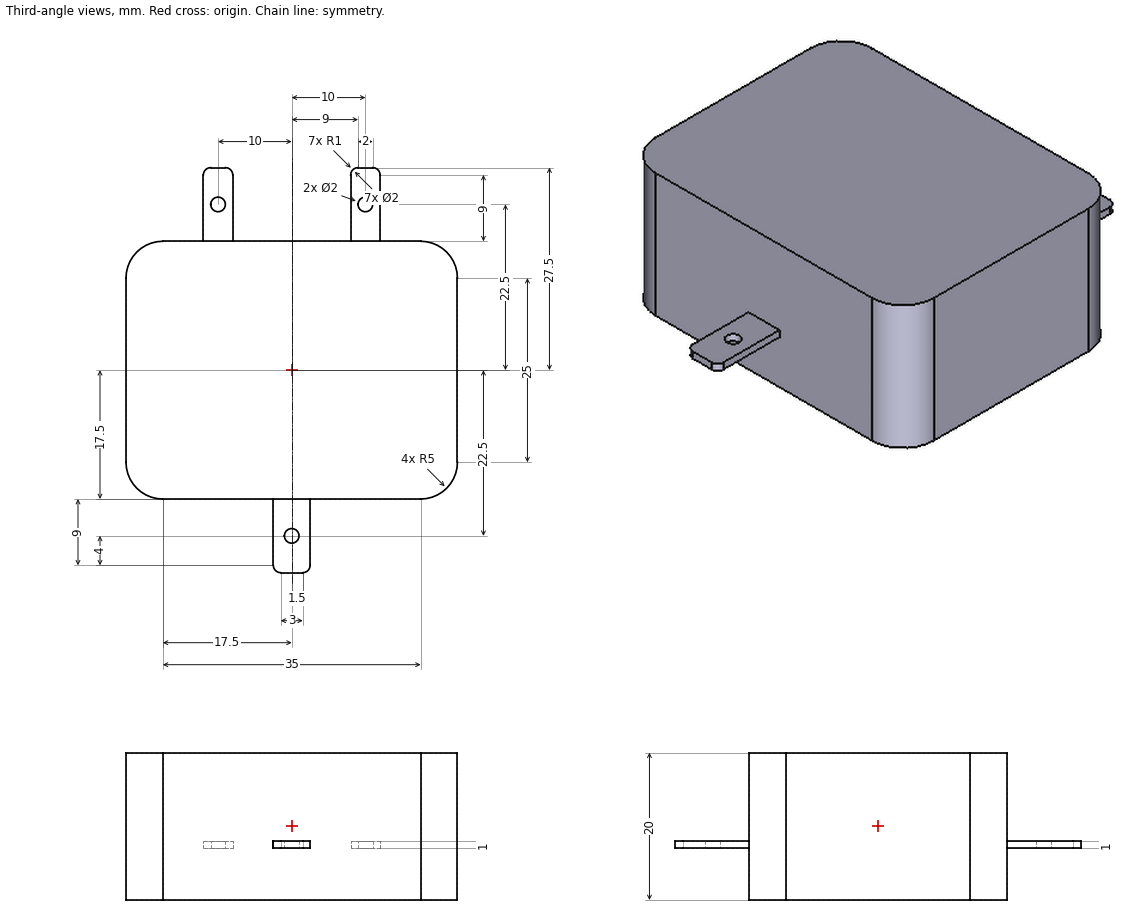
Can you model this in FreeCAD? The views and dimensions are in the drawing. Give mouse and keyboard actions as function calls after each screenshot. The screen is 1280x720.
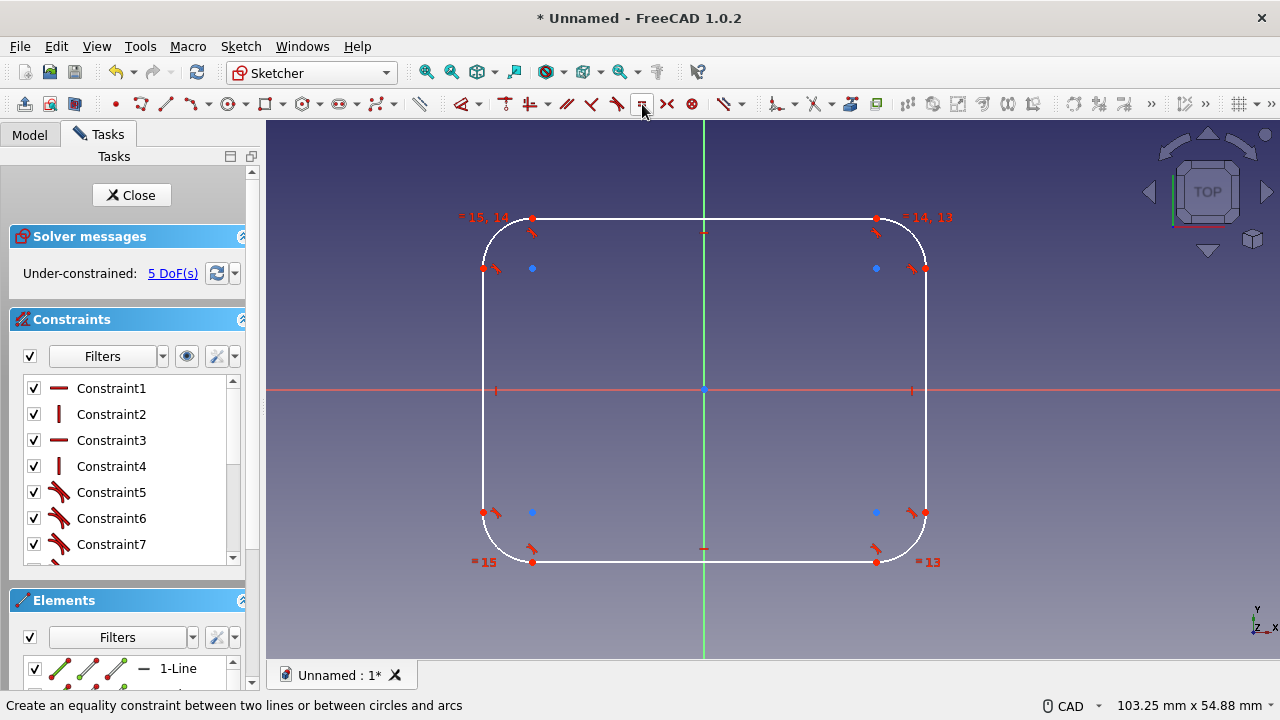
click(460, 104)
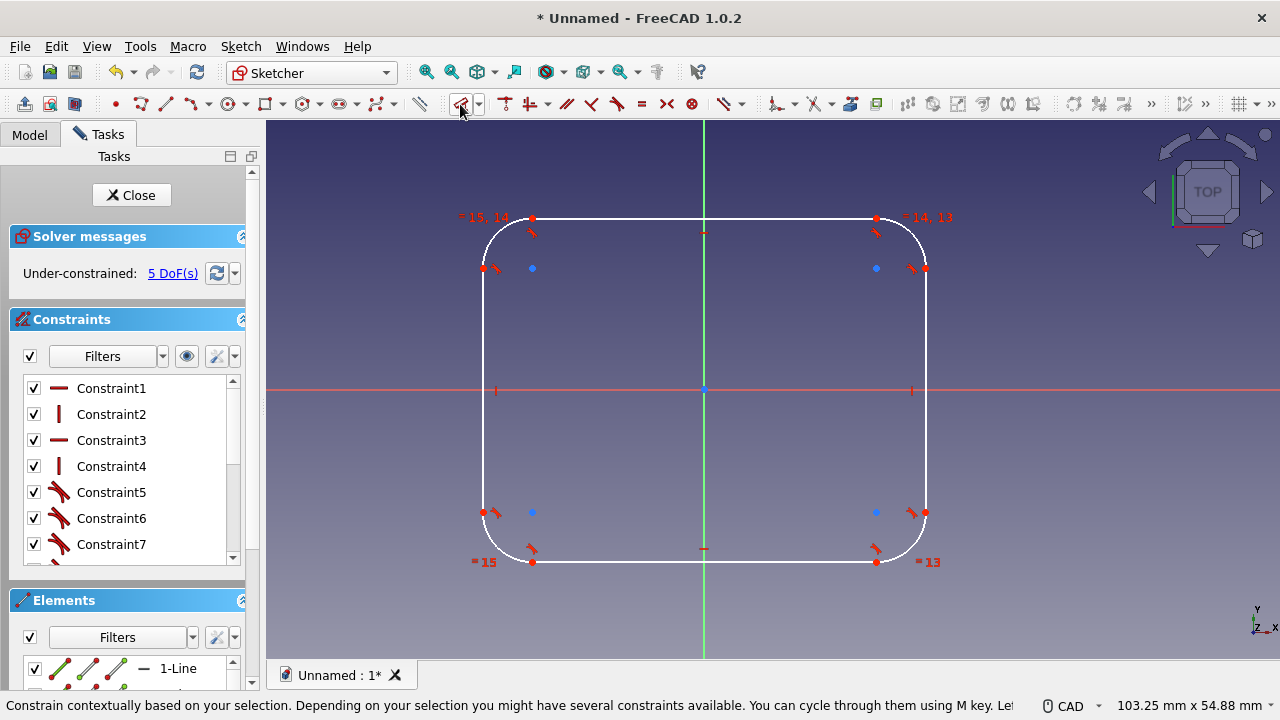
click(899, 557)
click(914, 586)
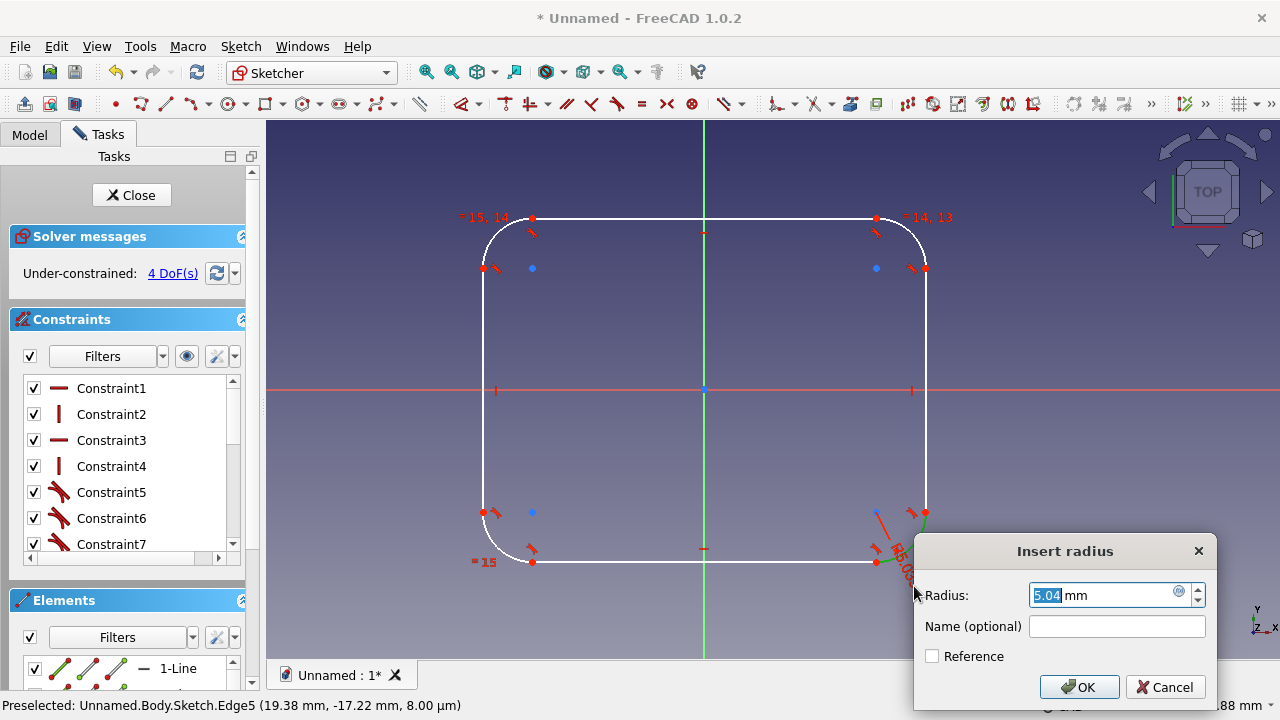
text(5)
key(Return)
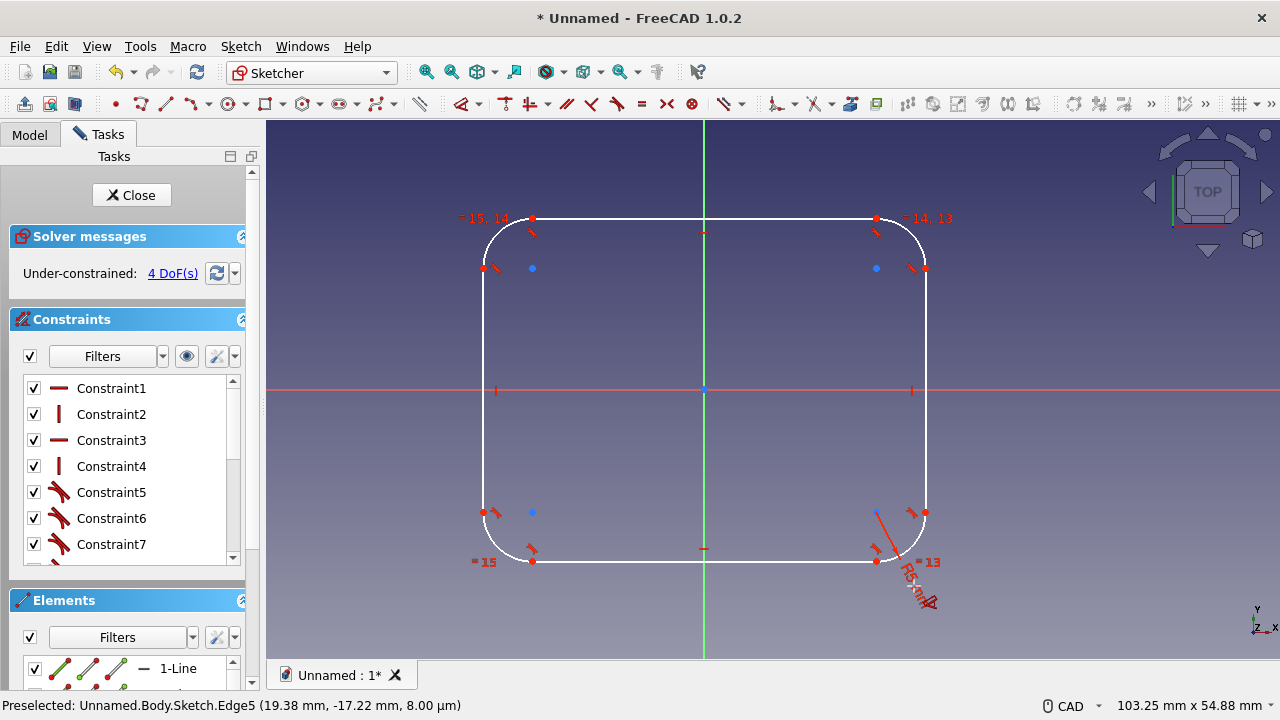
click(636, 562)
click(625, 596)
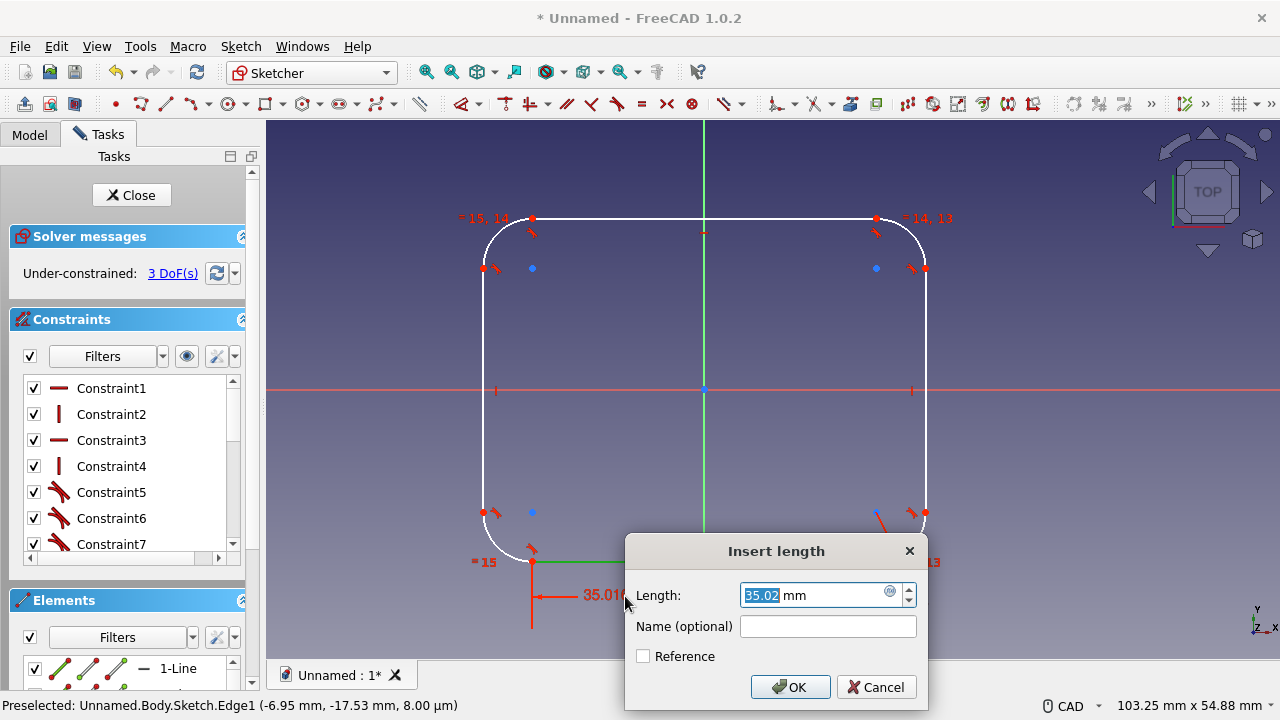
text(35)
key(Return)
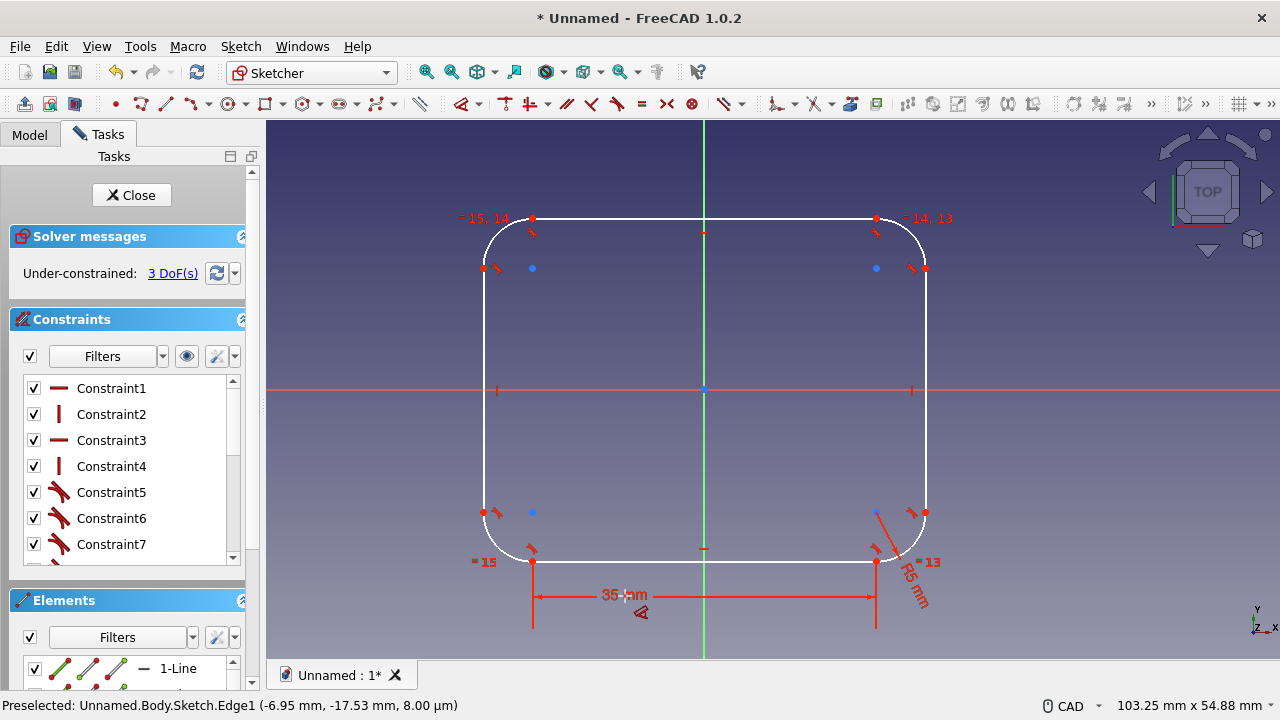
click(926, 439)
click(960, 334)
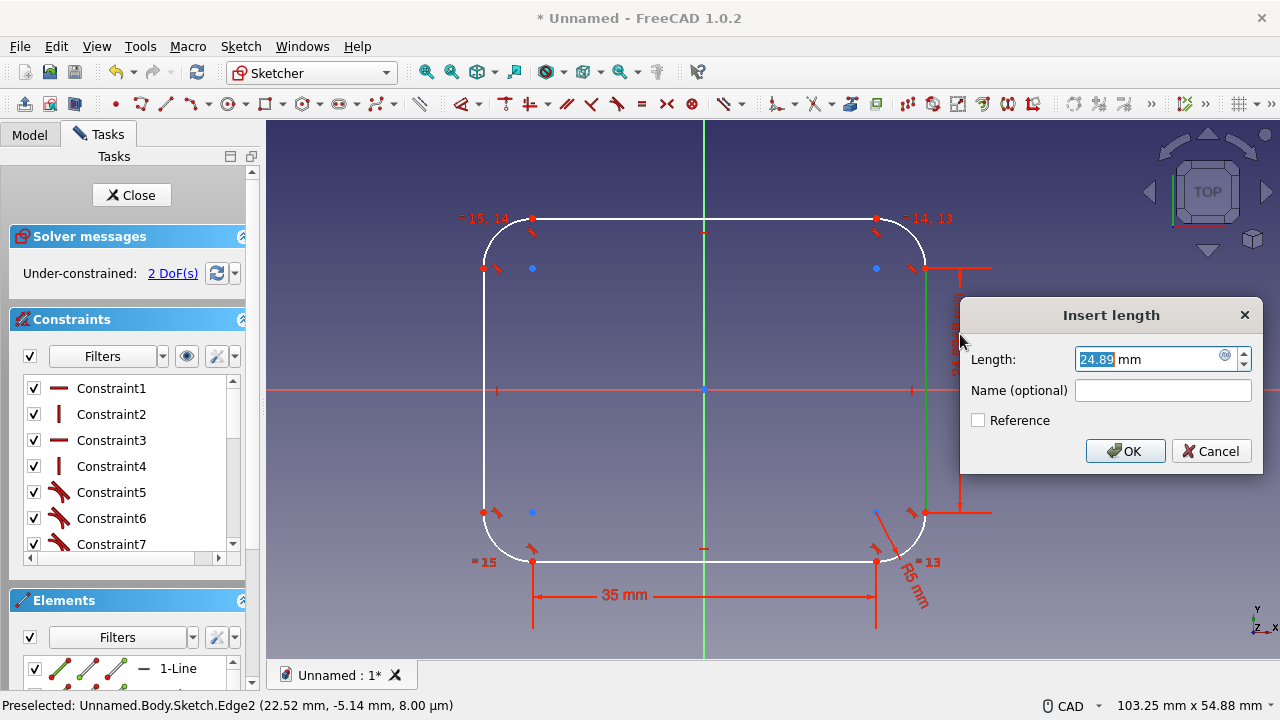
text(25)
key(Return)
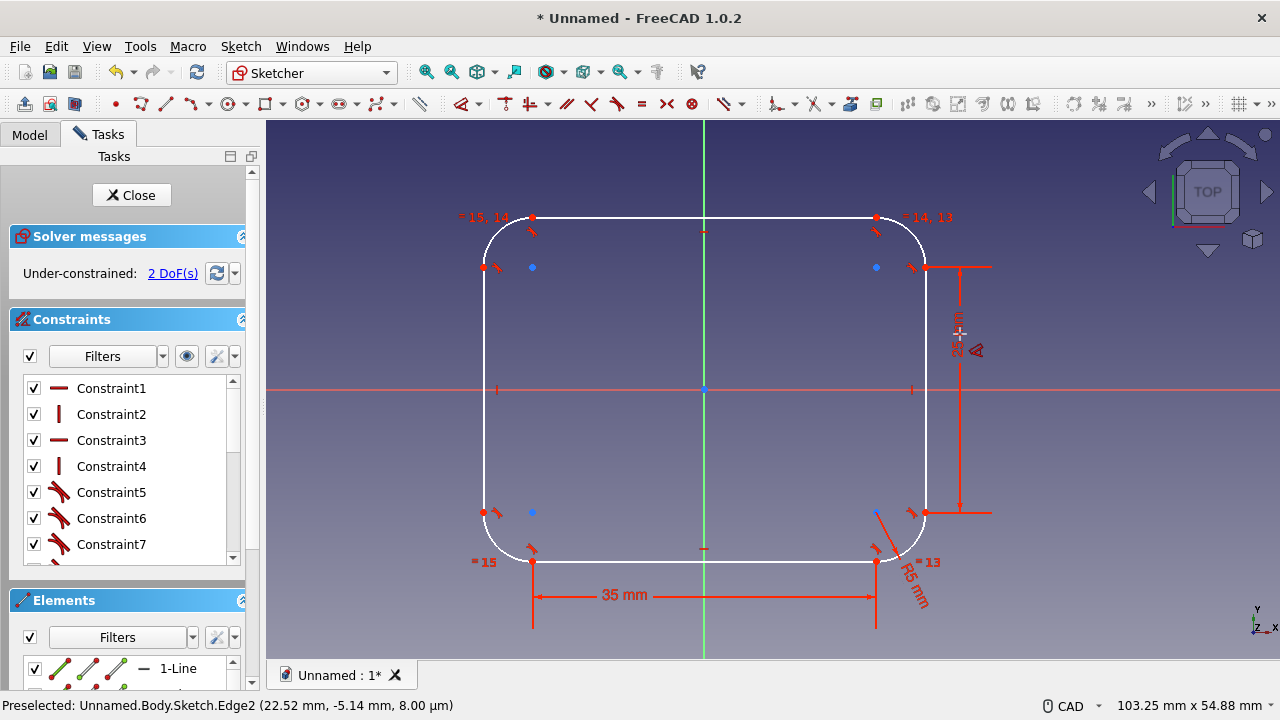
click(533, 562)
click(618, 356)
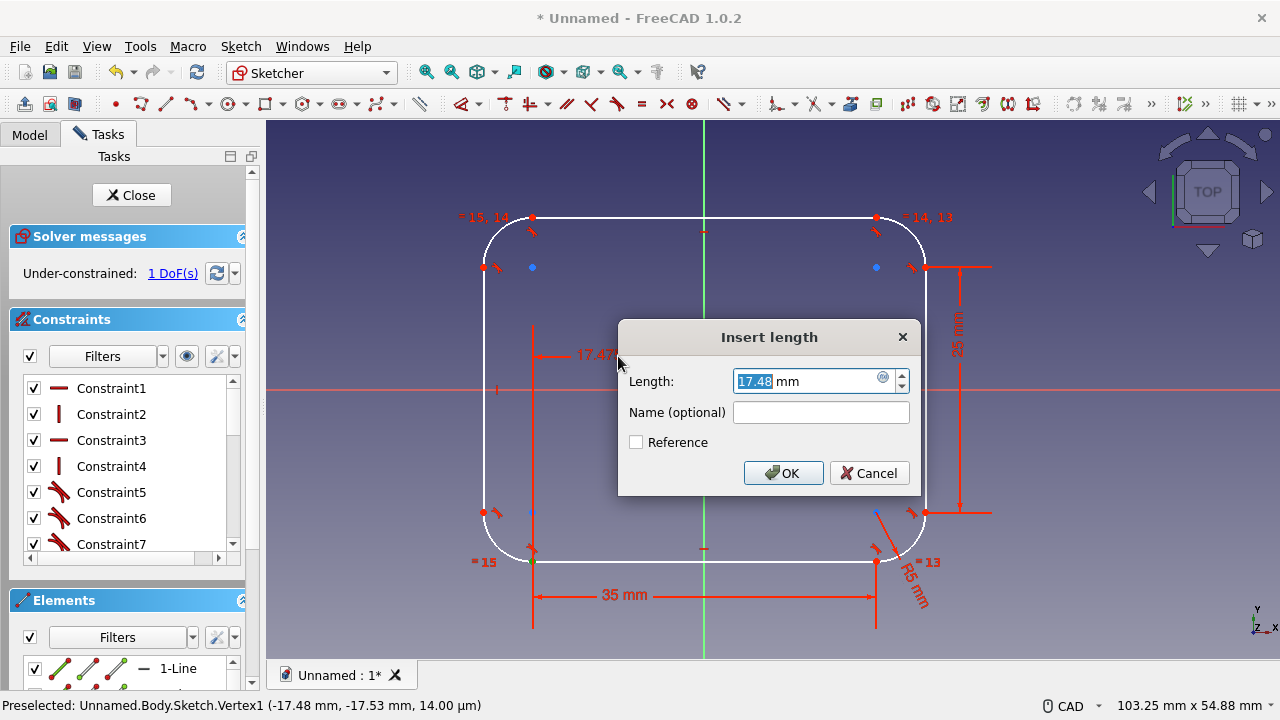
text(17.5)
key(Return)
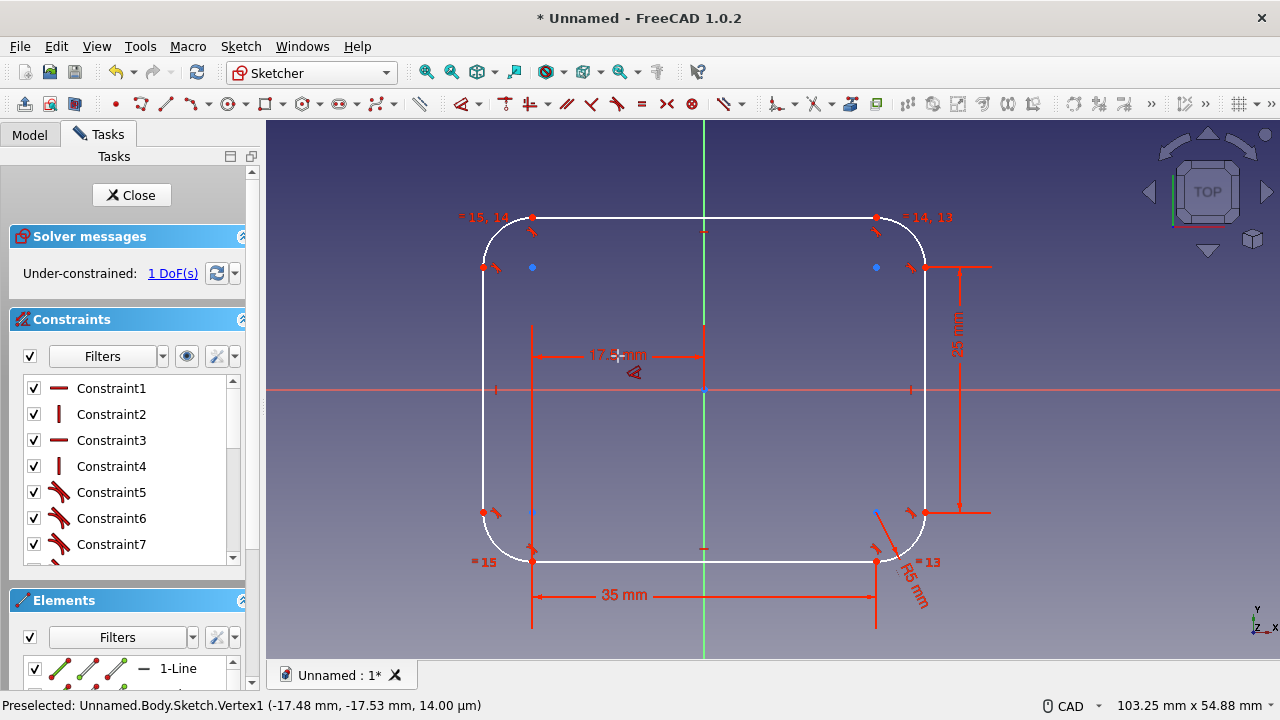
click(532, 562)
click(498, 476)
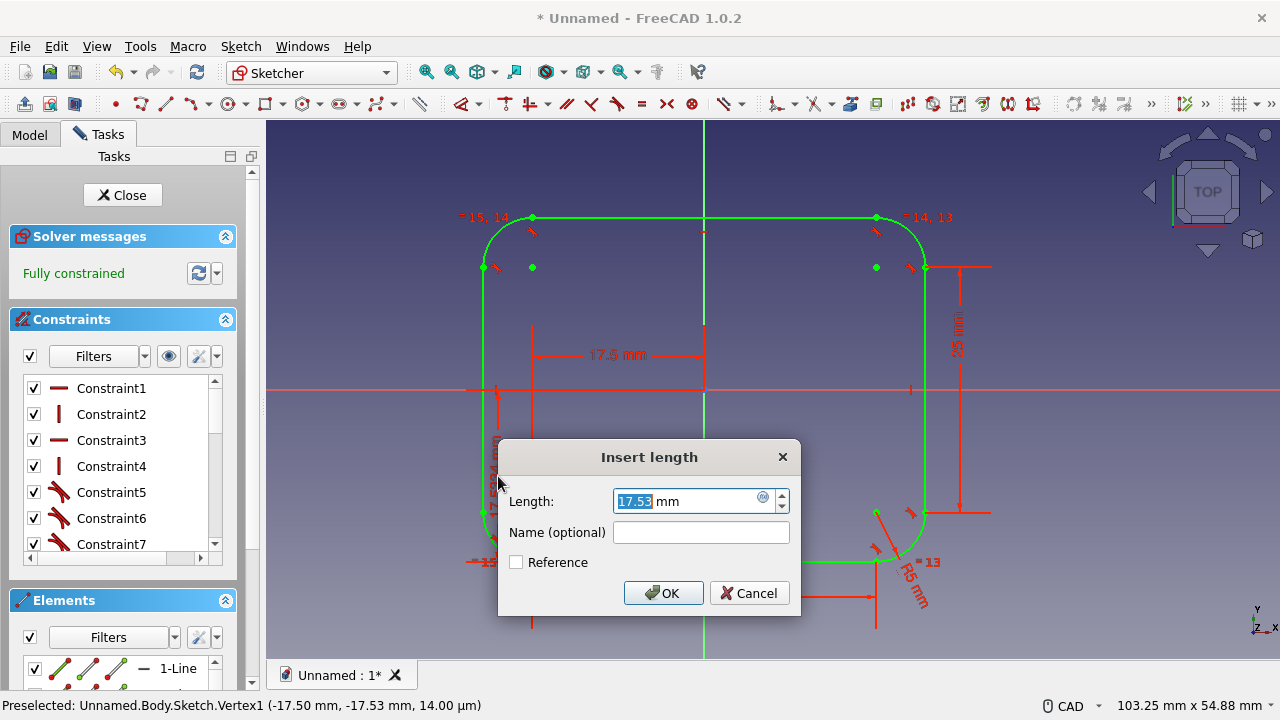
text(17.5)
key(Return)
key(Escape)